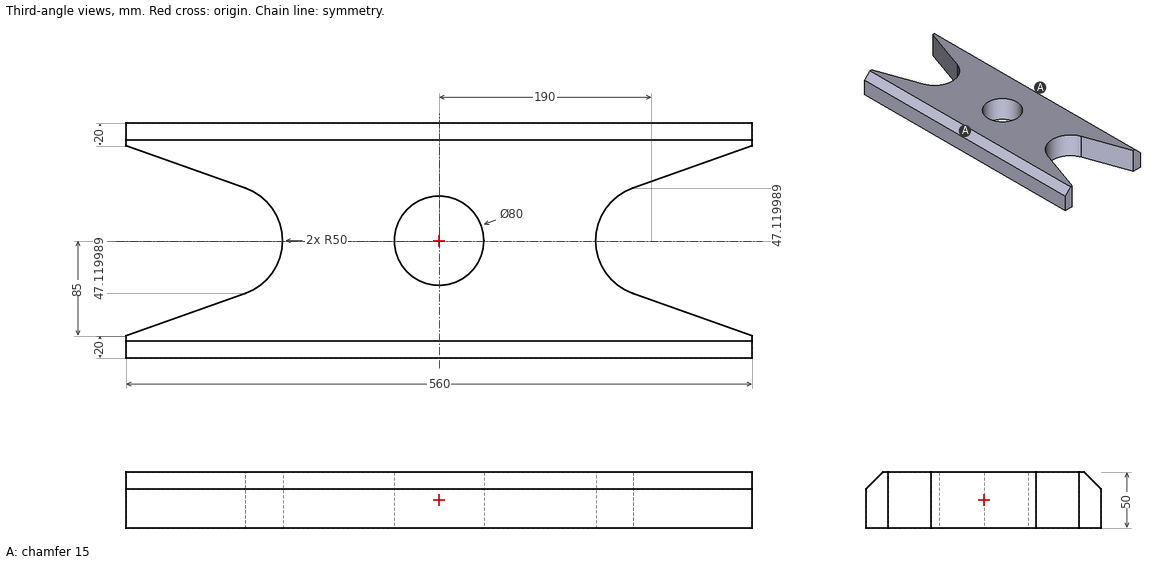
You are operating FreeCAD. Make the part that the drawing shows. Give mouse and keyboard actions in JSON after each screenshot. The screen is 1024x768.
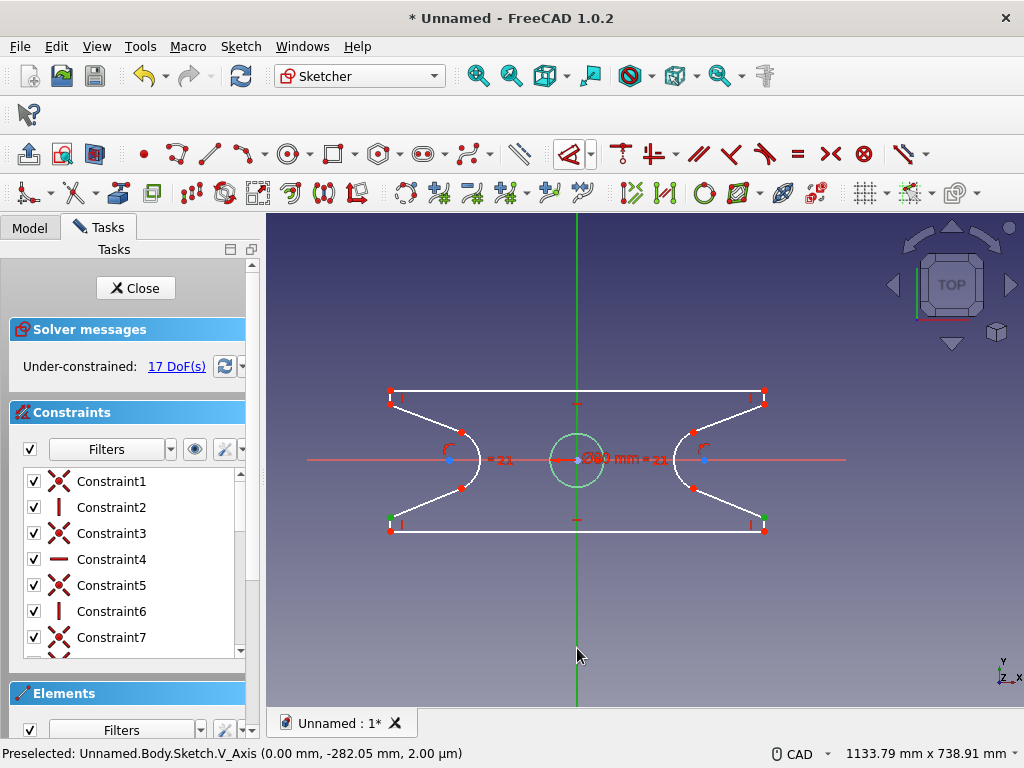
{"action": "key", "text": "s"}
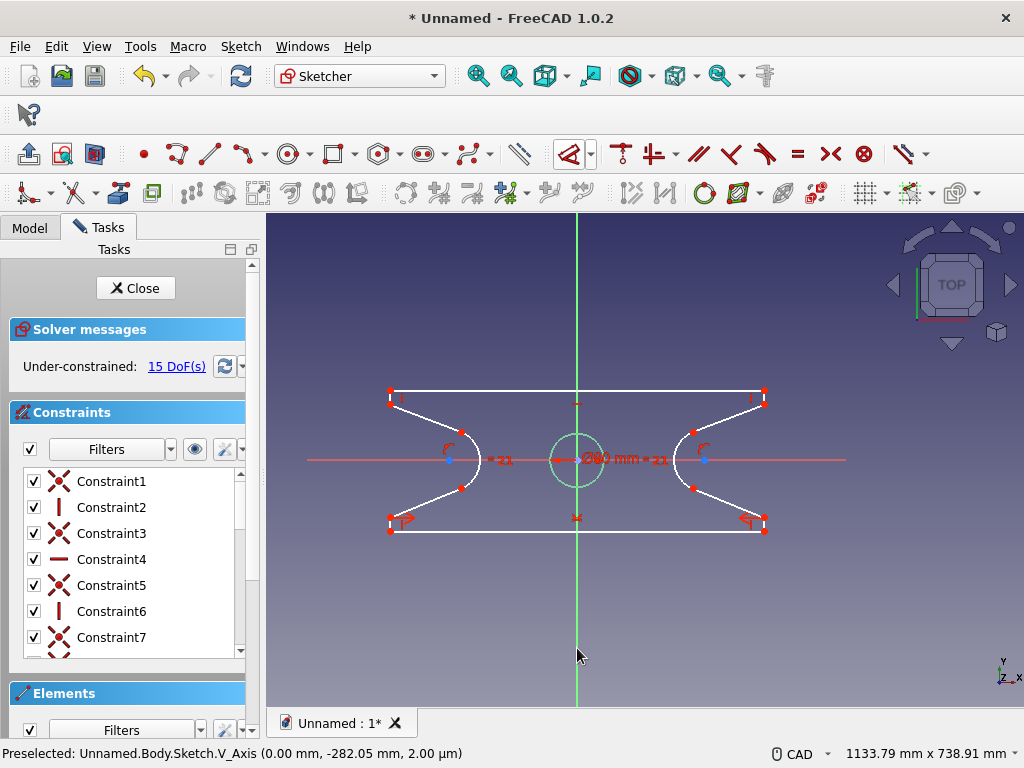
{"action": "left_click", "coordinate": [461, 489]}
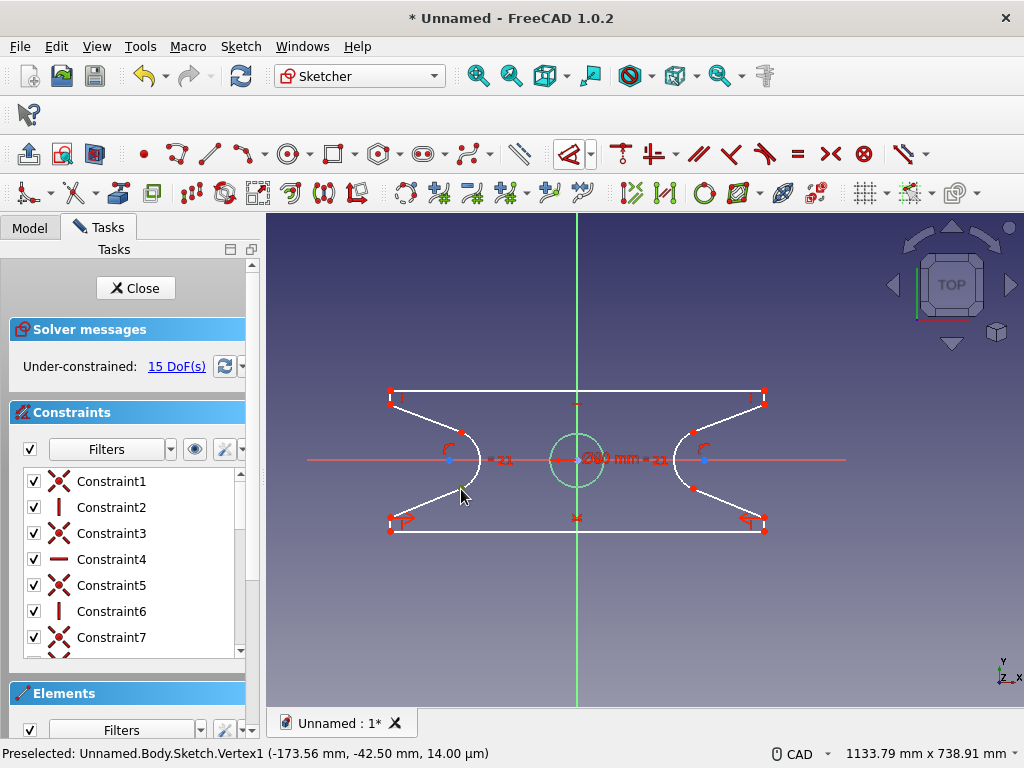
{"action": "left_click", "coordinate": [693, 489]}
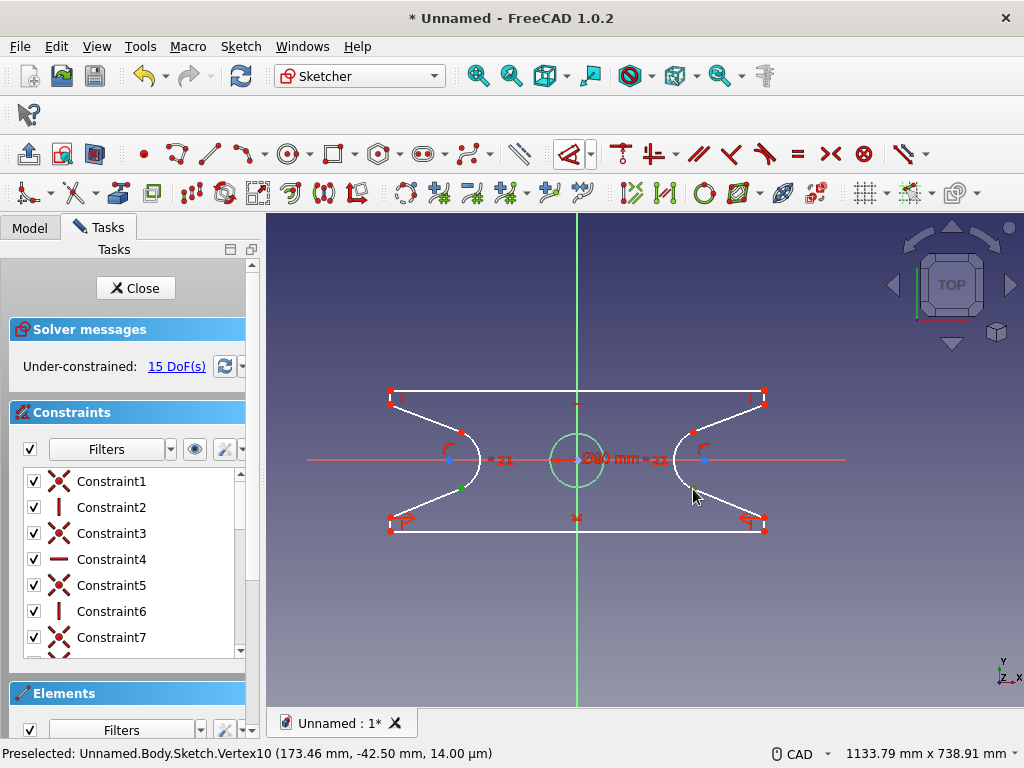
{"action": "left_click", "coordinate": [577, 648]}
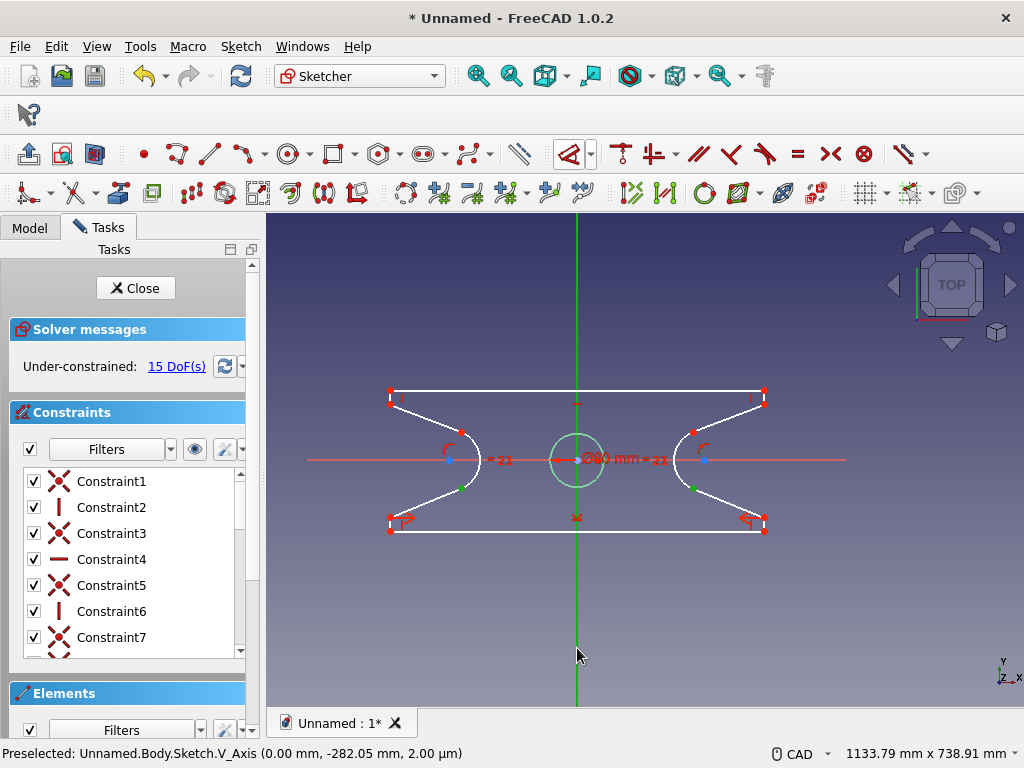
{"action": "key", "text": "s"}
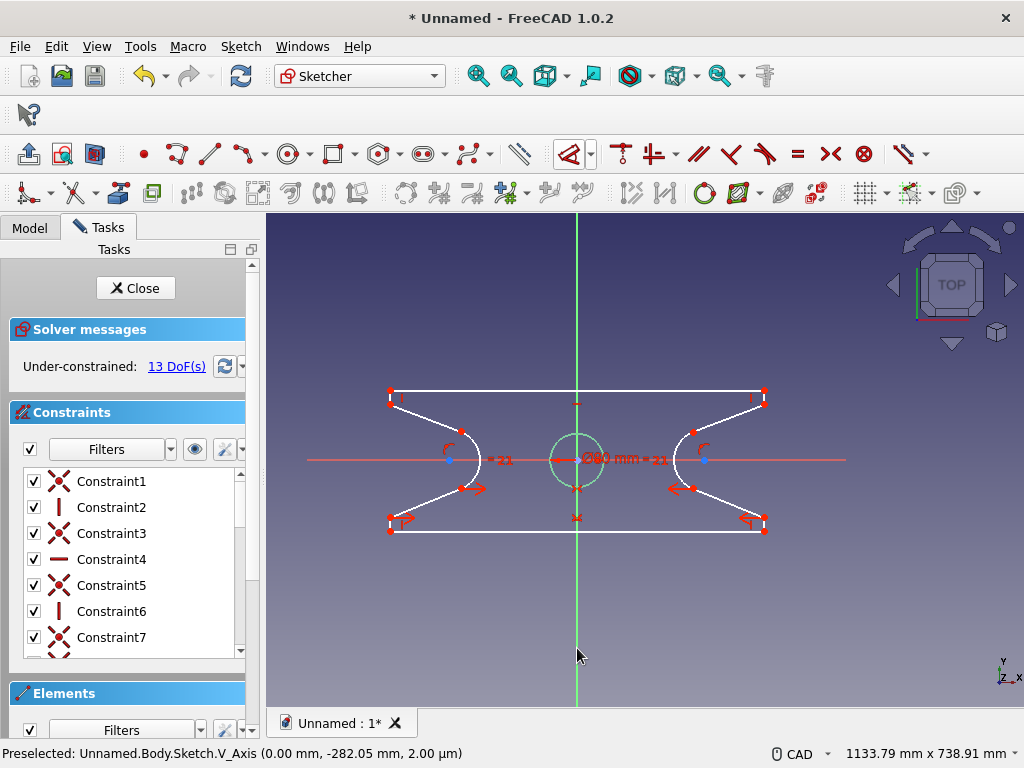
{"action": "left_click", "coordinate": [764, 518]}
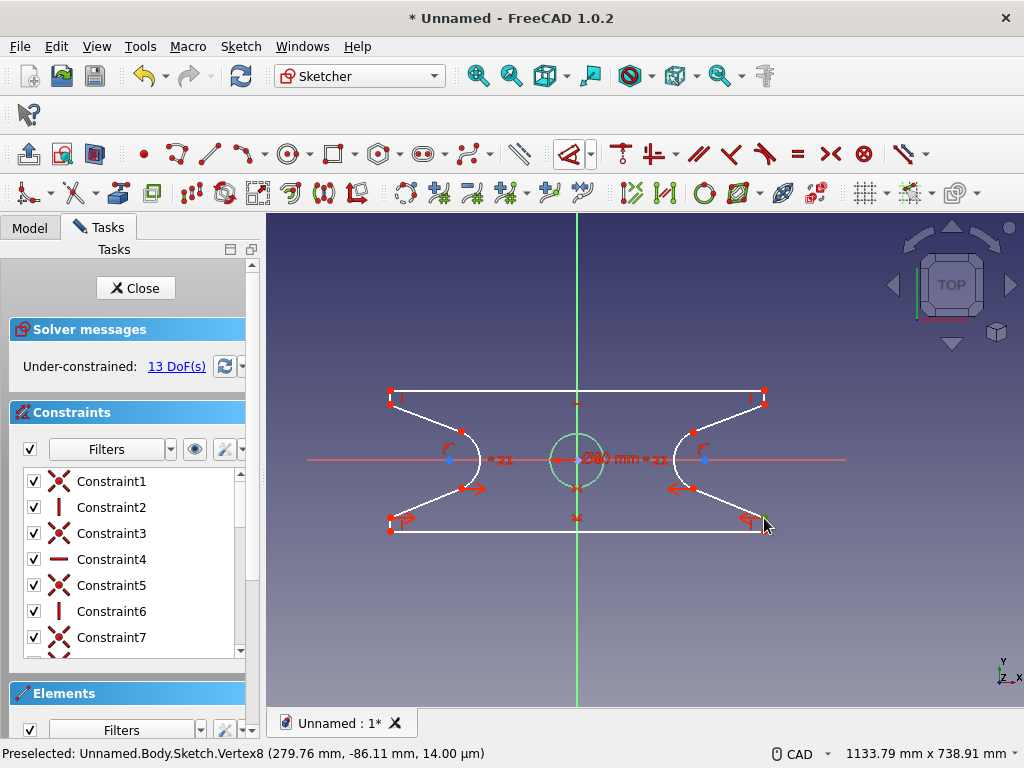
{"action": "left_click", "coordinate": [764, 405]}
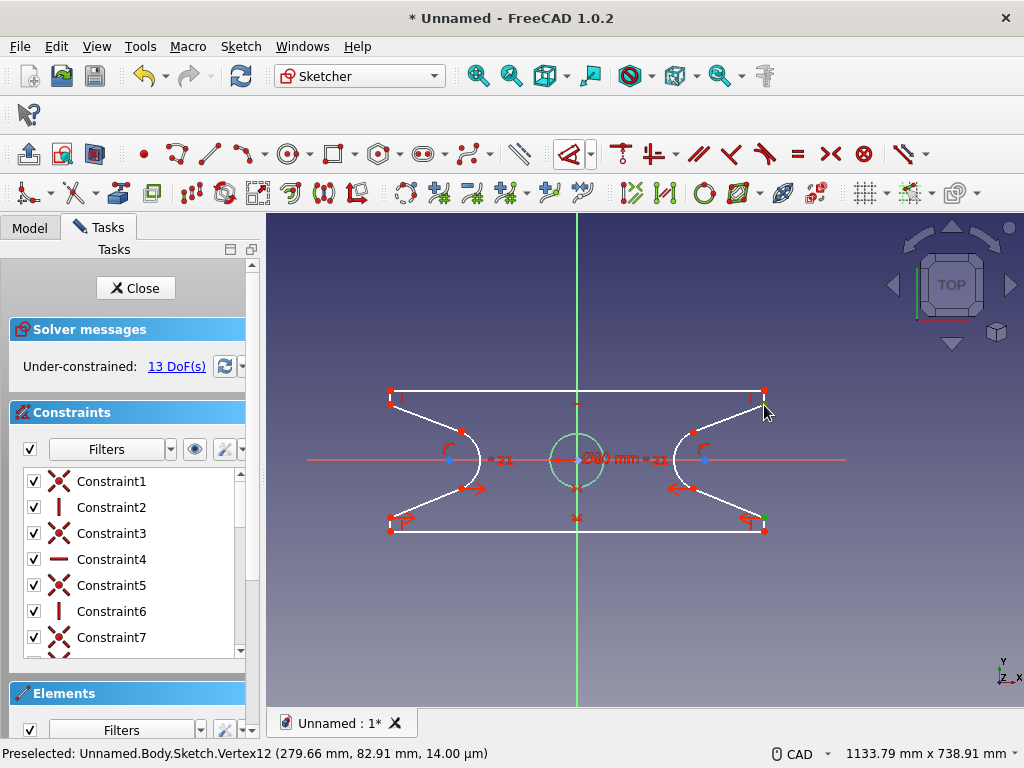
{"action": "left_click", "coordinate": [334, 460]}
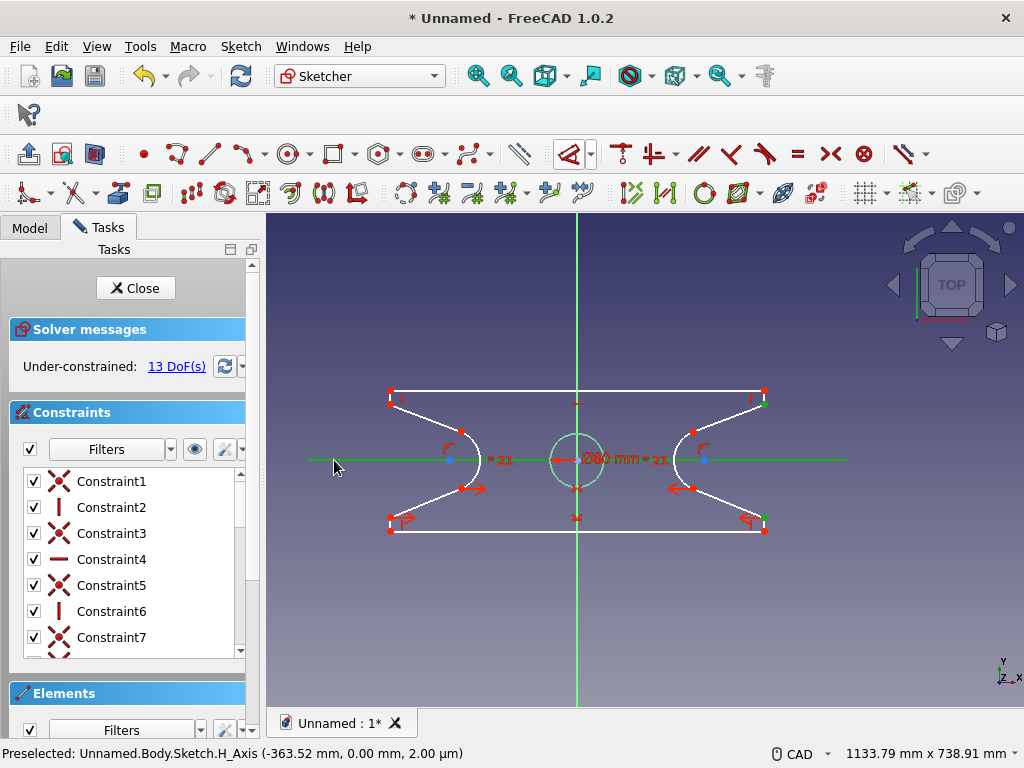
{"action": "key", "text": "s"}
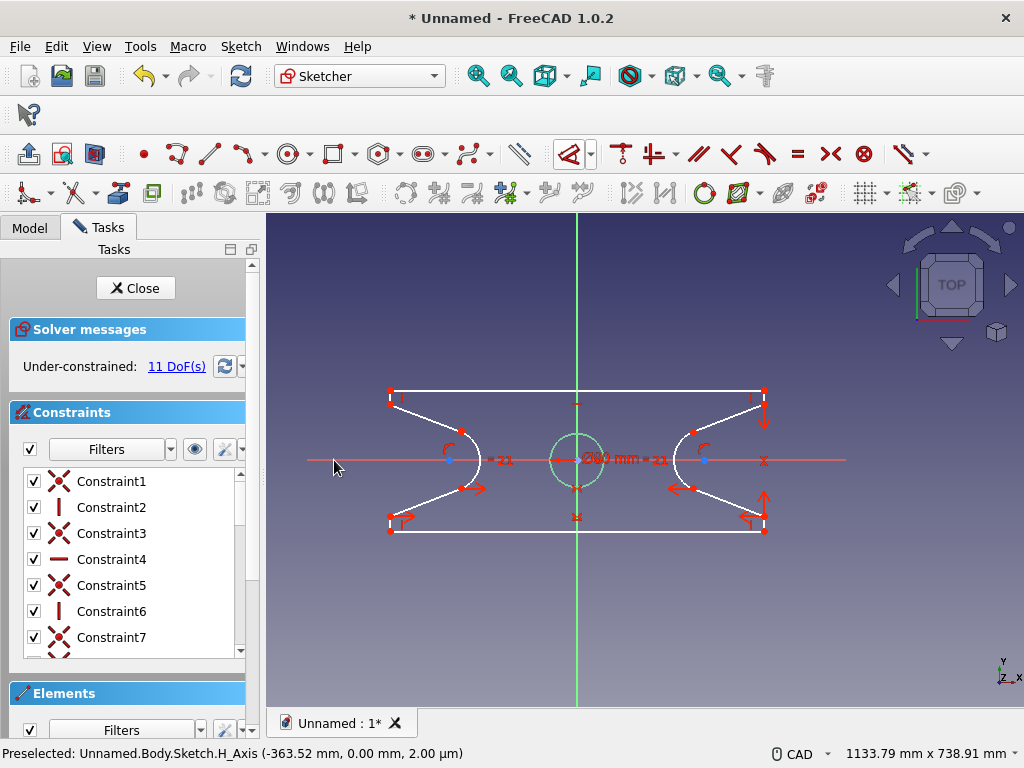
{"action": "left_click", "coordinate": [390, 532]}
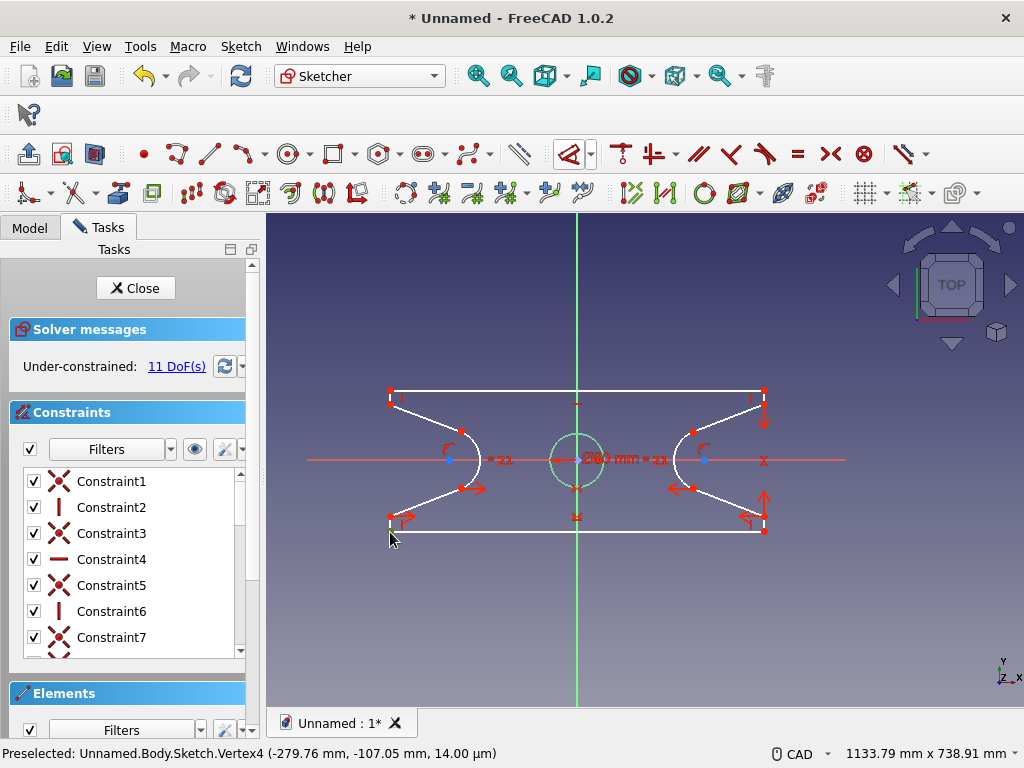
{"action": "left_click", "coordinate": [390, 391]}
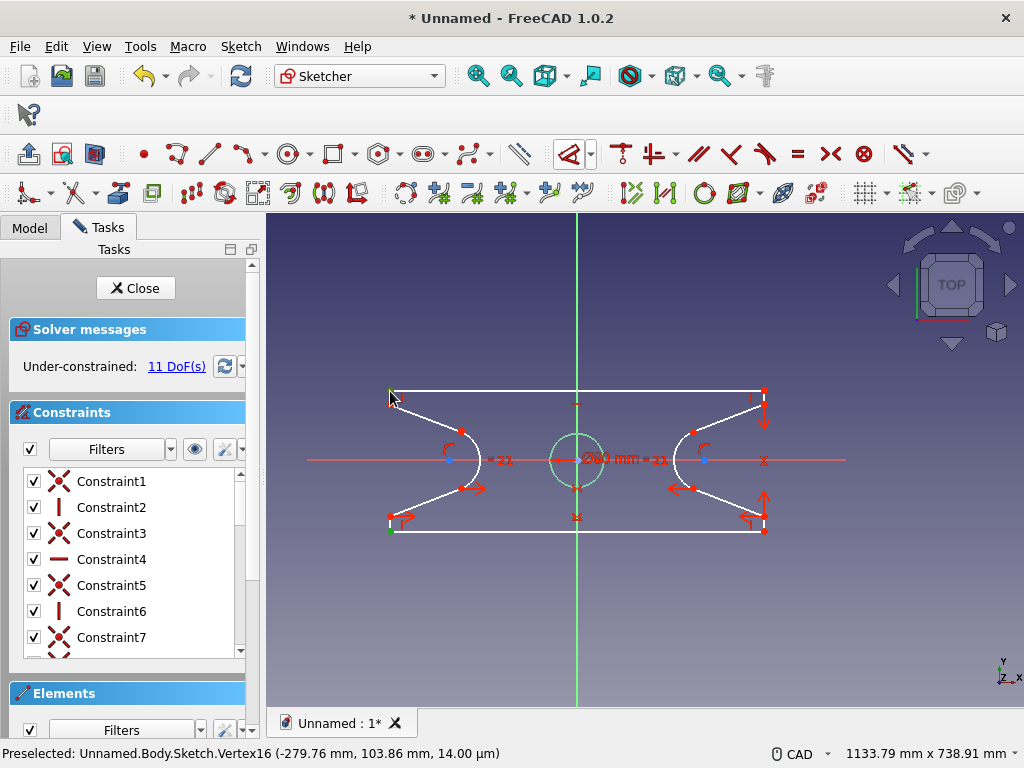
{"action": "left_click", "coordinate": [334, 460]}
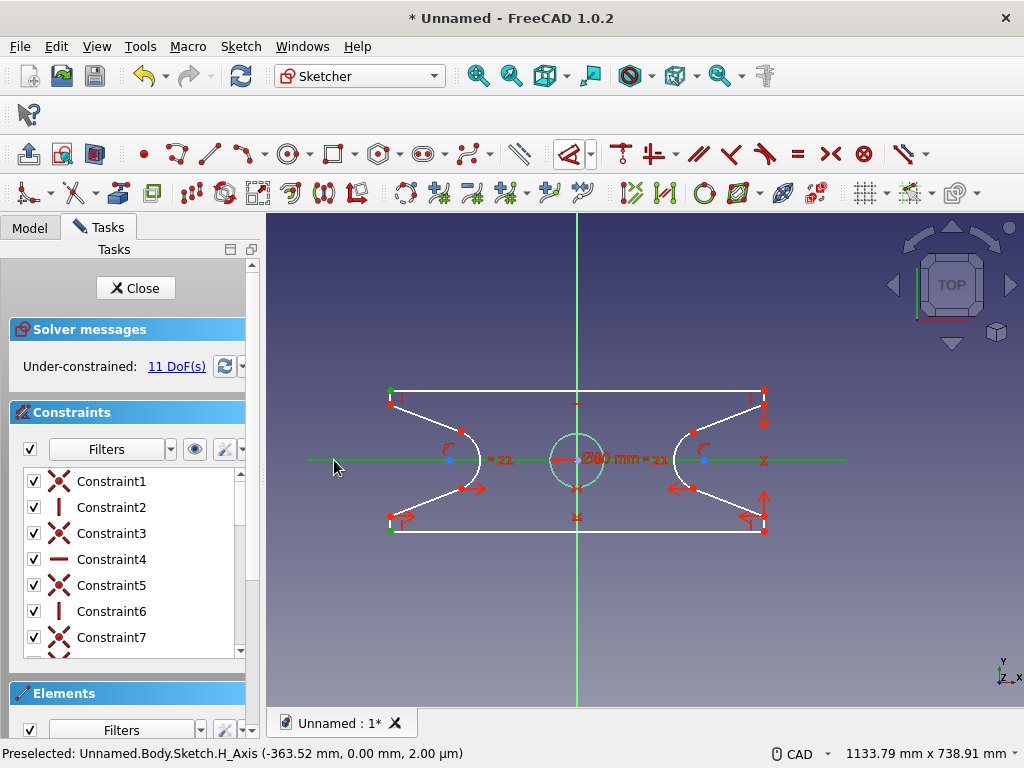
{"action": "left_click", "coordinate": [831, 154]}